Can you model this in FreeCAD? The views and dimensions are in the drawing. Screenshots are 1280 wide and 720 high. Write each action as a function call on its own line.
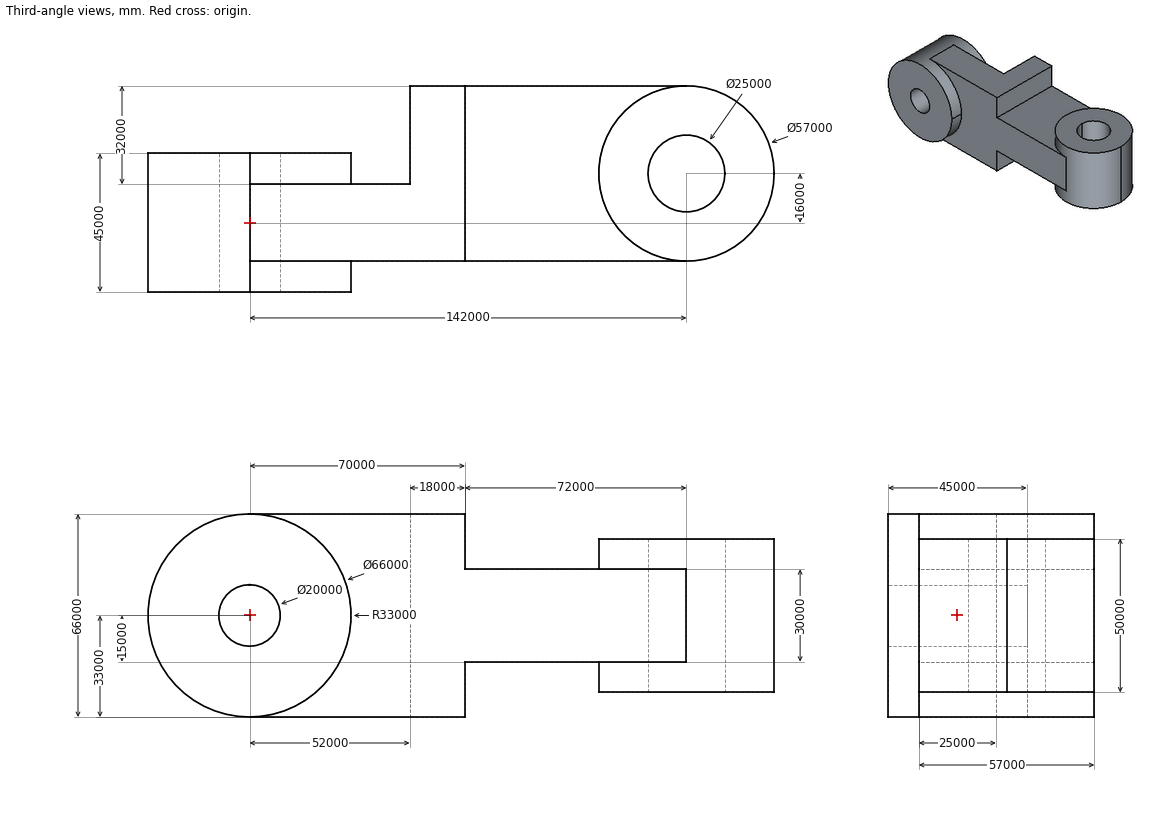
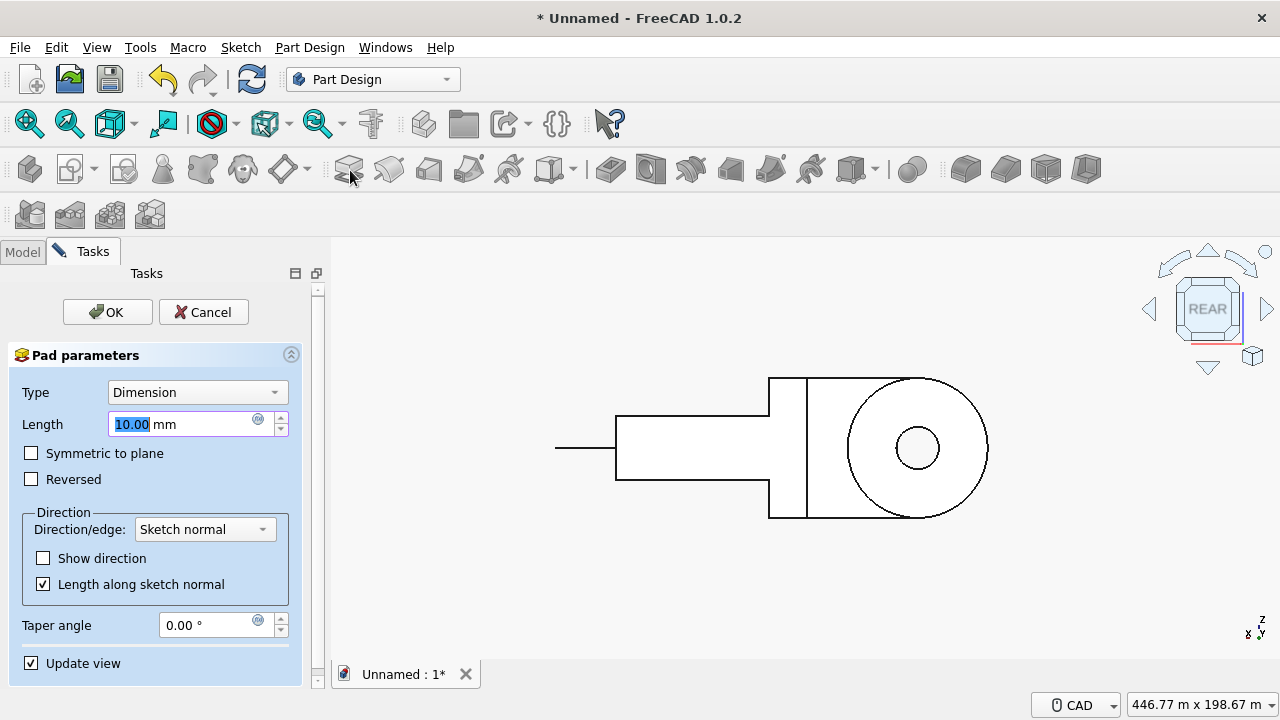
text(50000)
key(Tab)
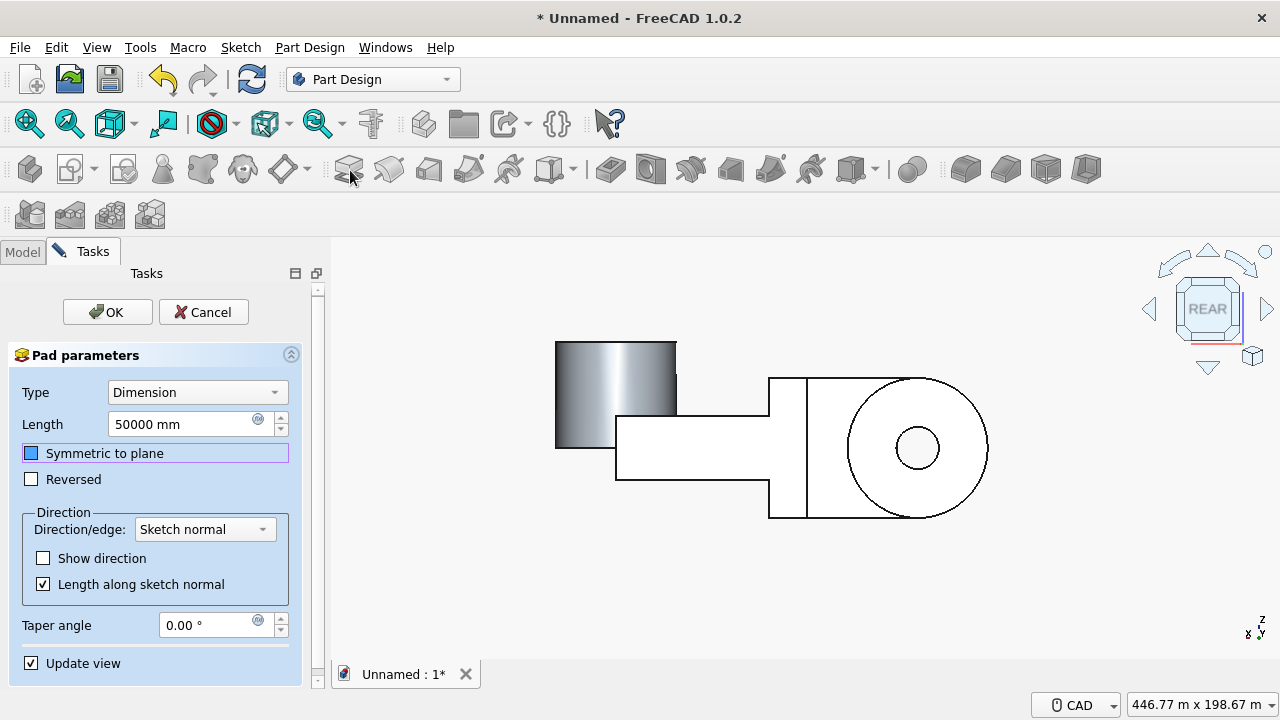
click(30, 453)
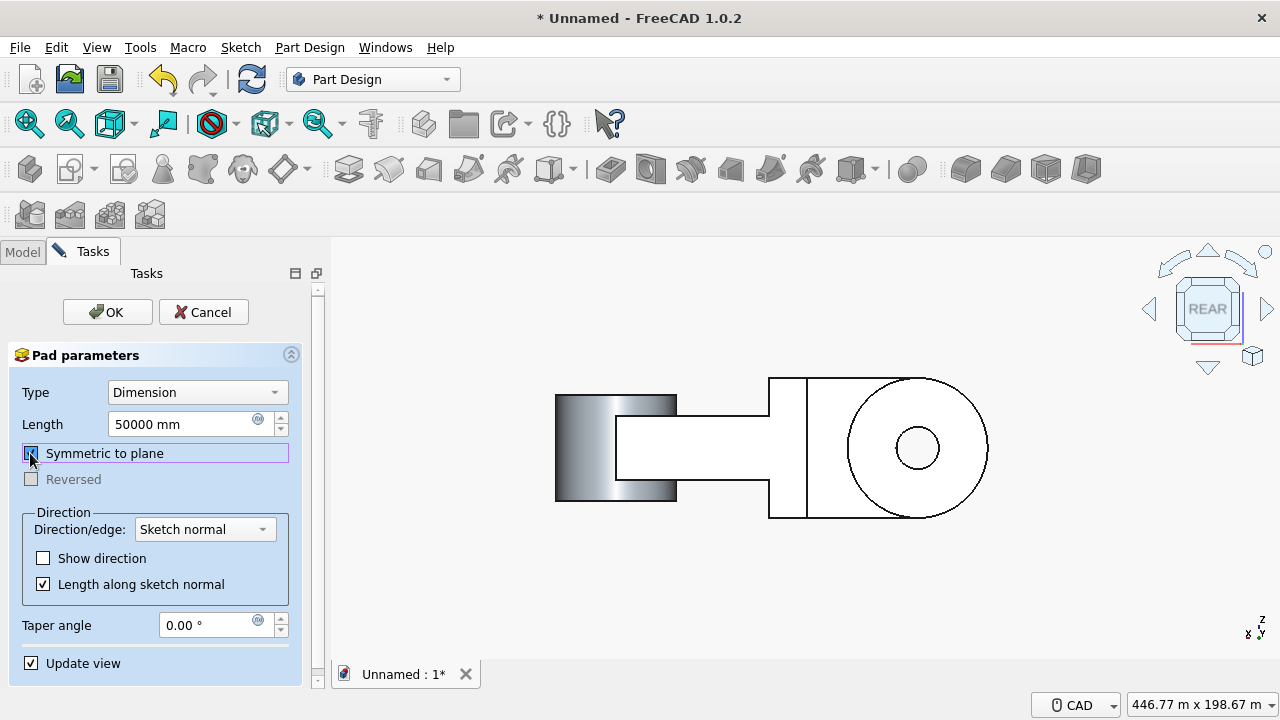
click(108, 312)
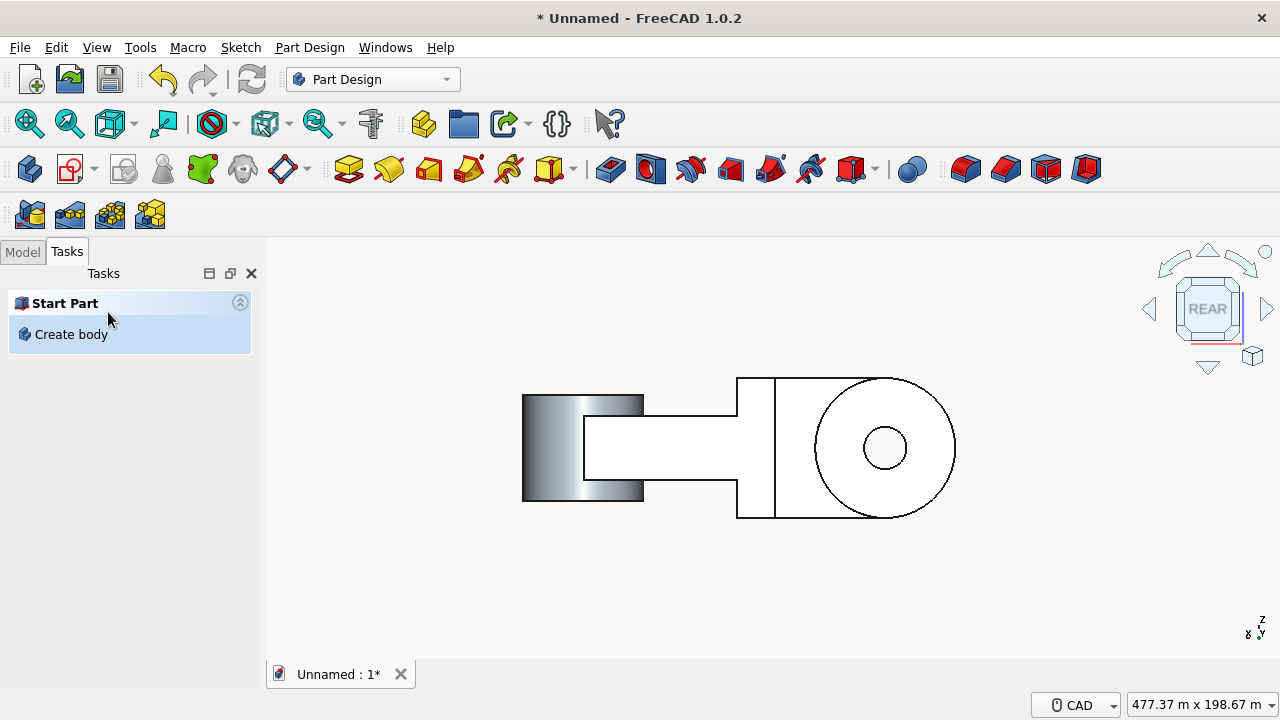
key(v)
key(f)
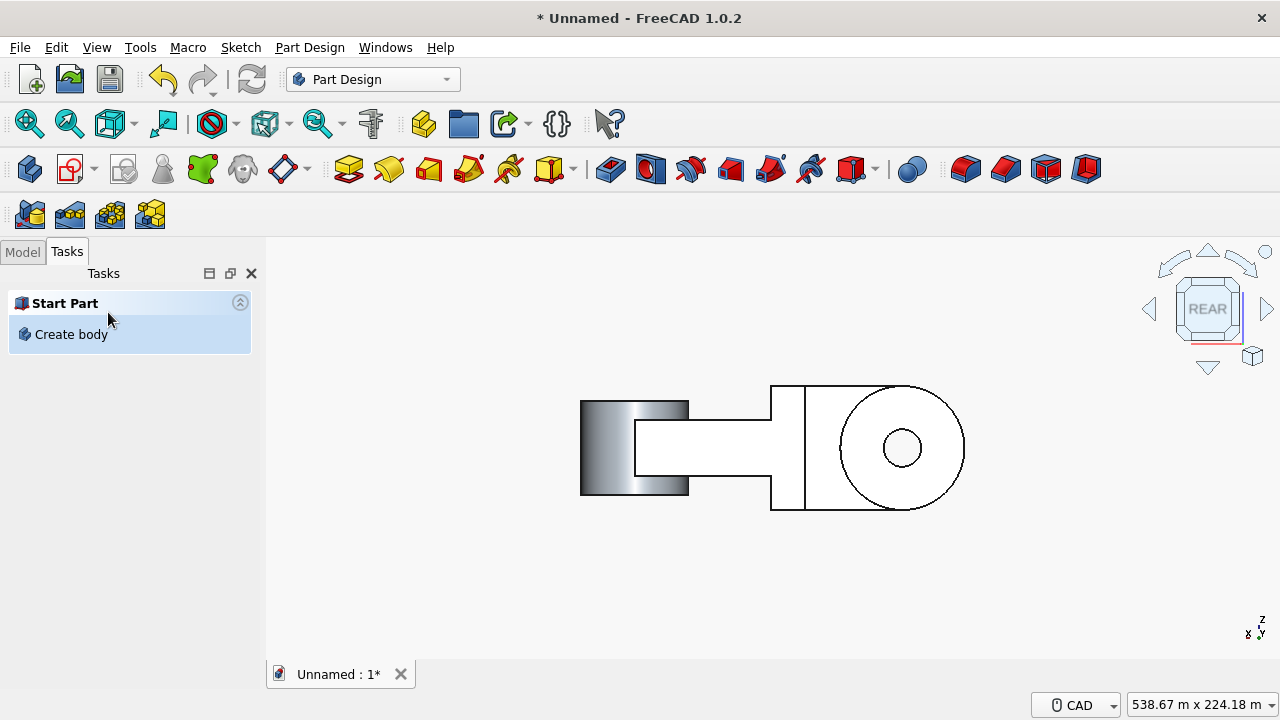
key(0)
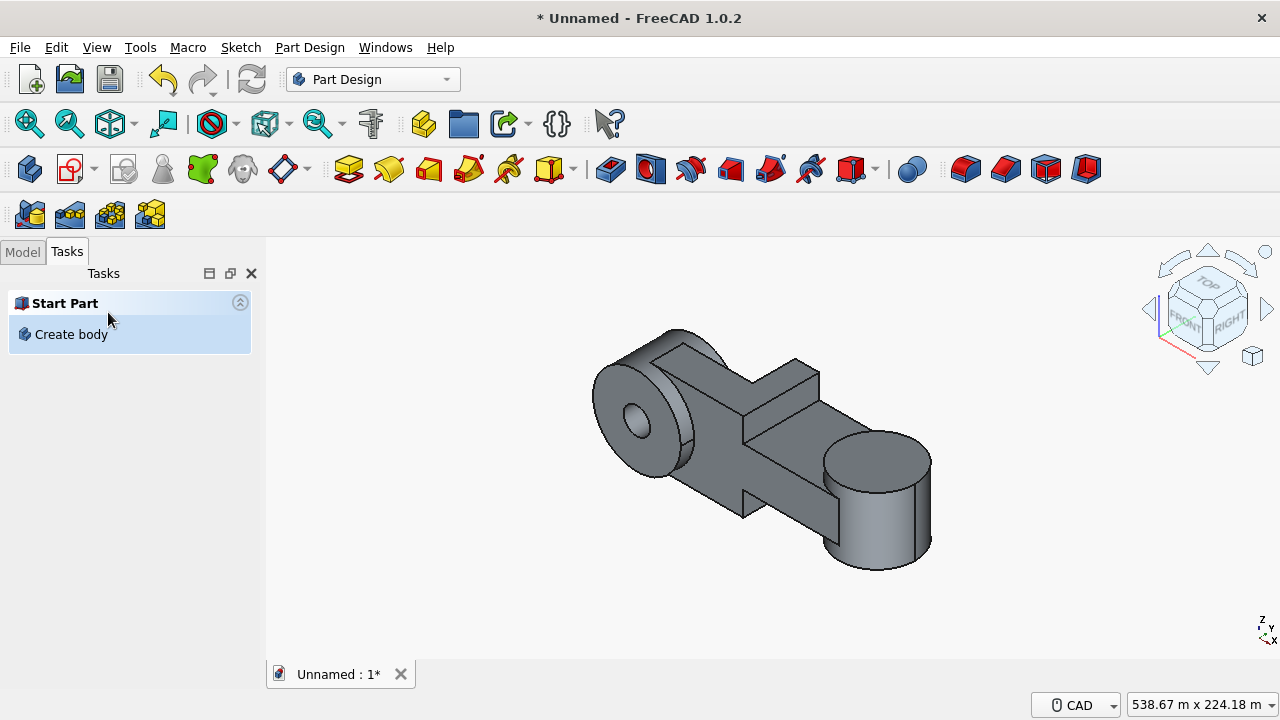
click(877, 461)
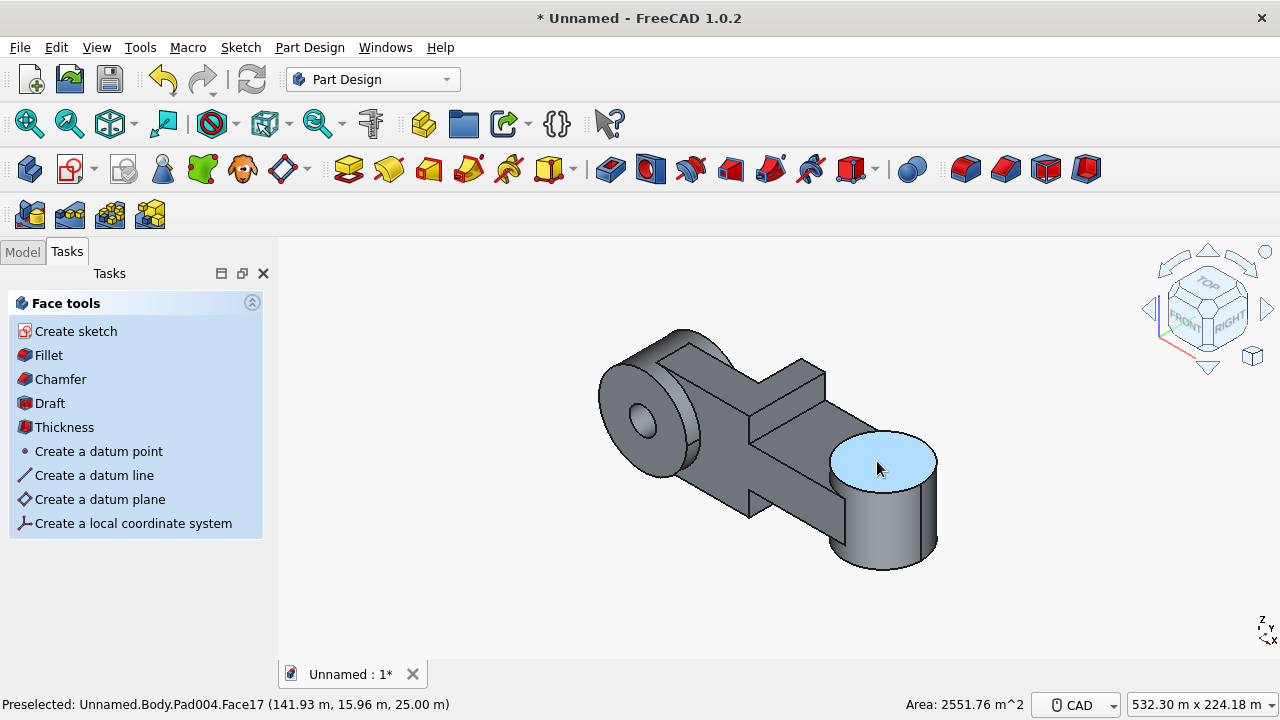
click(70, 170)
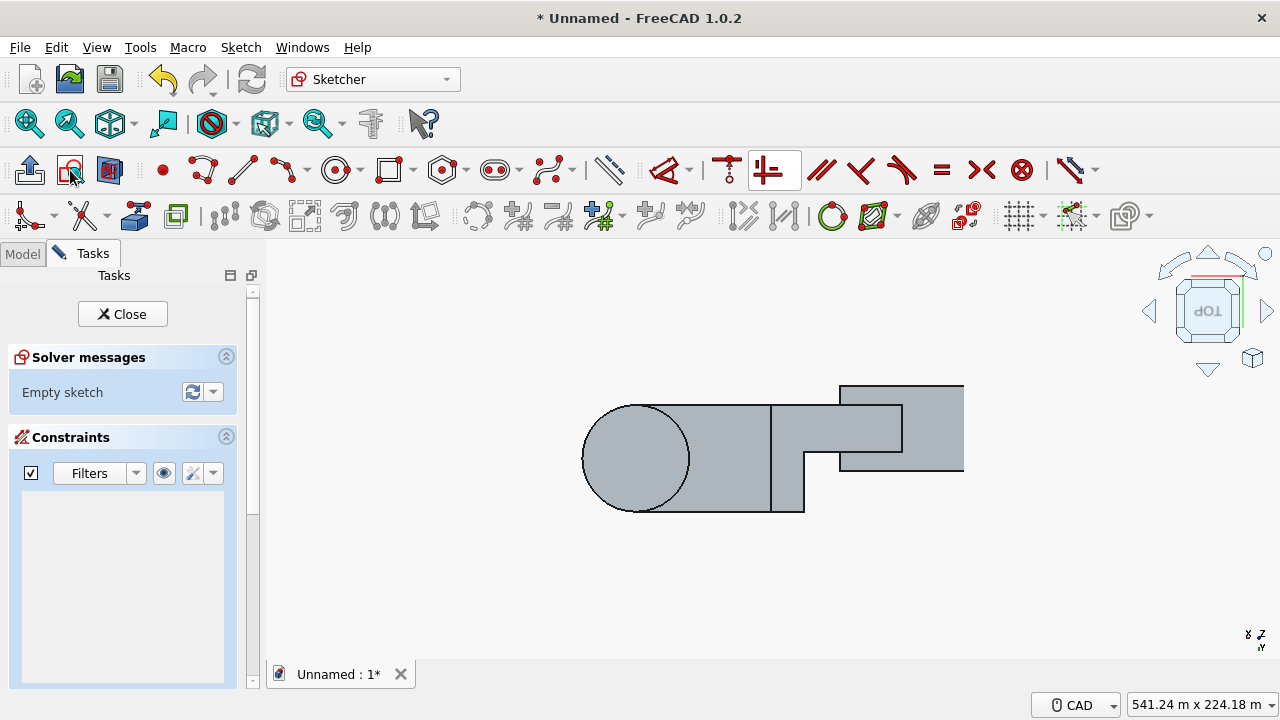
click(110, 170)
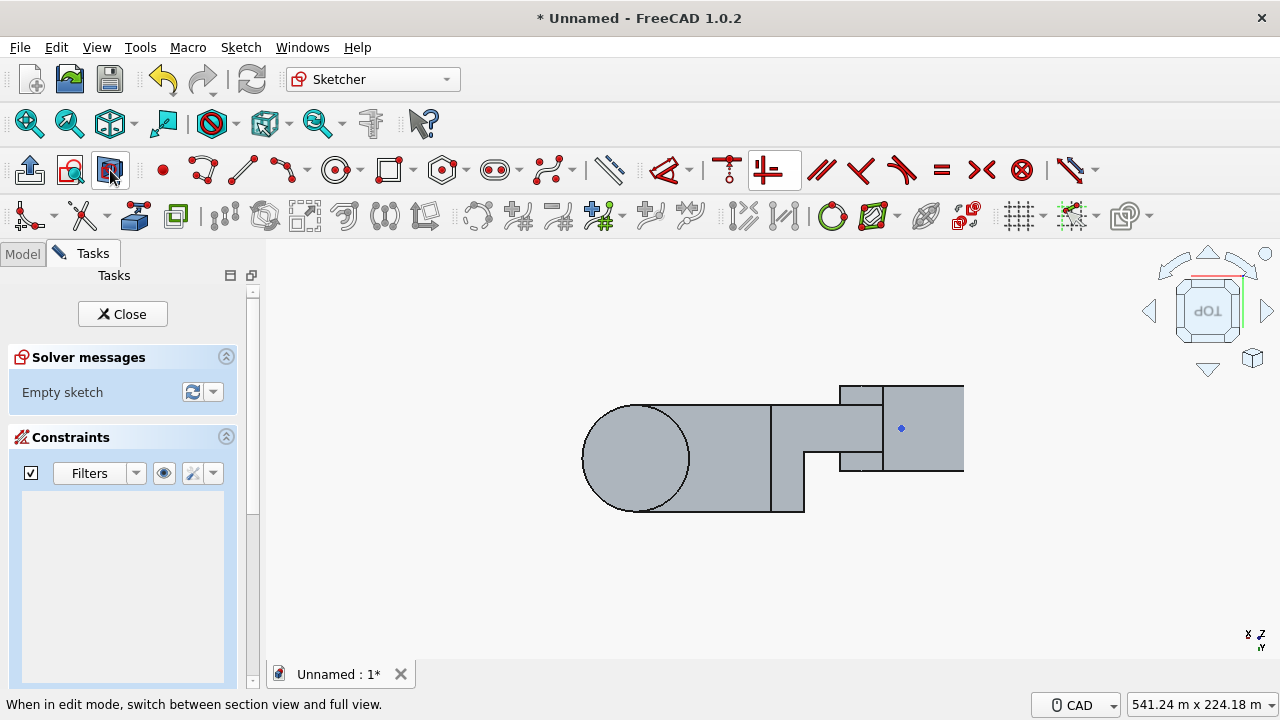
scroll(622, 460, up, 9)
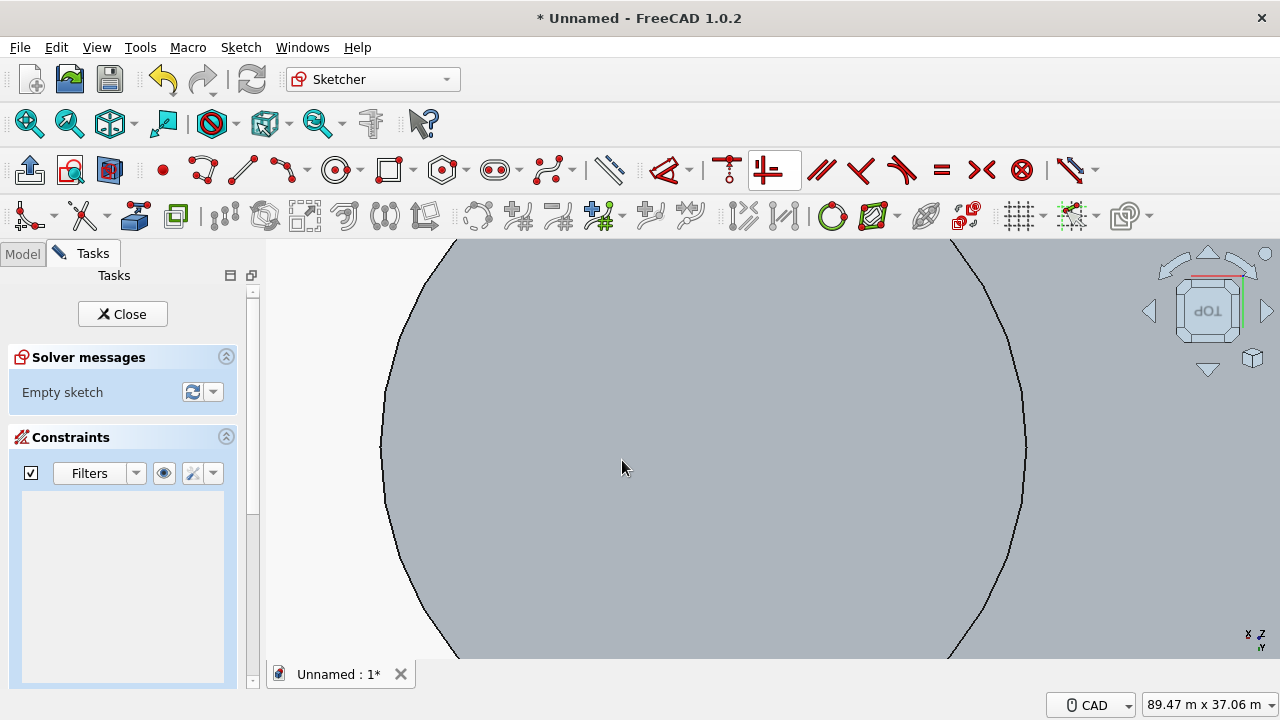
key(g)
key(c)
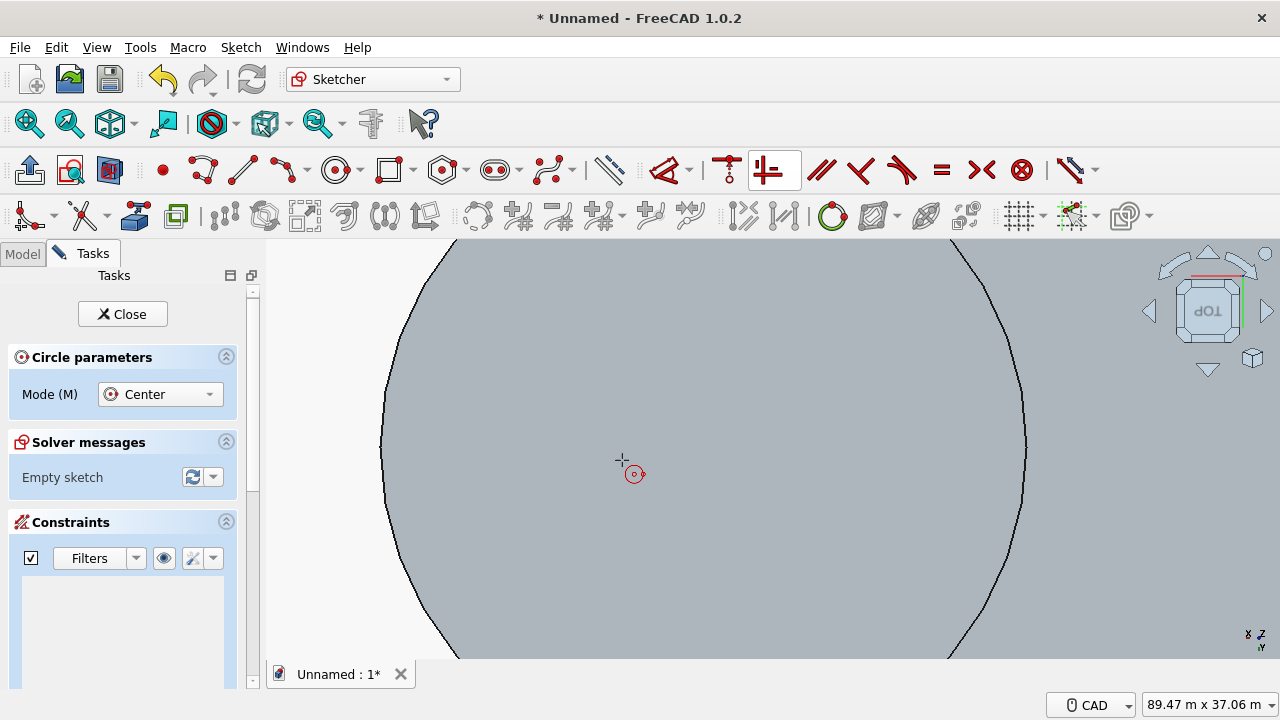
click(704, 447)
click(804, 347)
key(Escape)